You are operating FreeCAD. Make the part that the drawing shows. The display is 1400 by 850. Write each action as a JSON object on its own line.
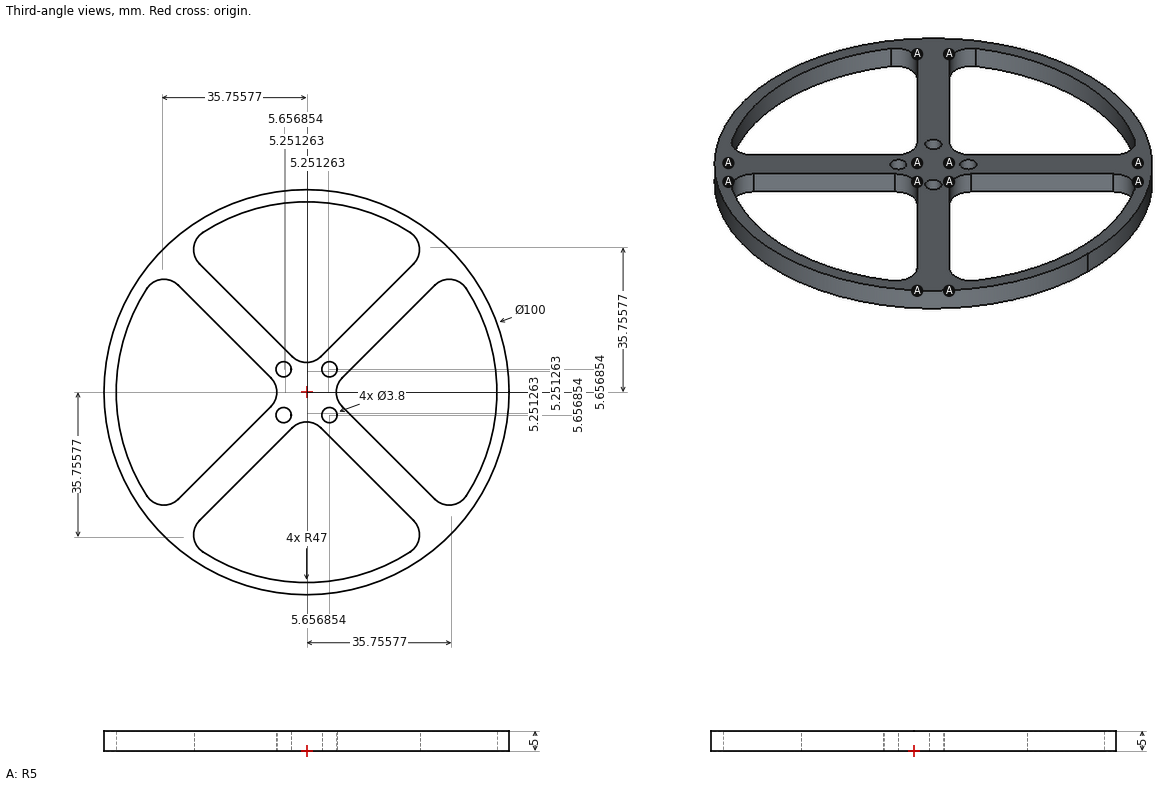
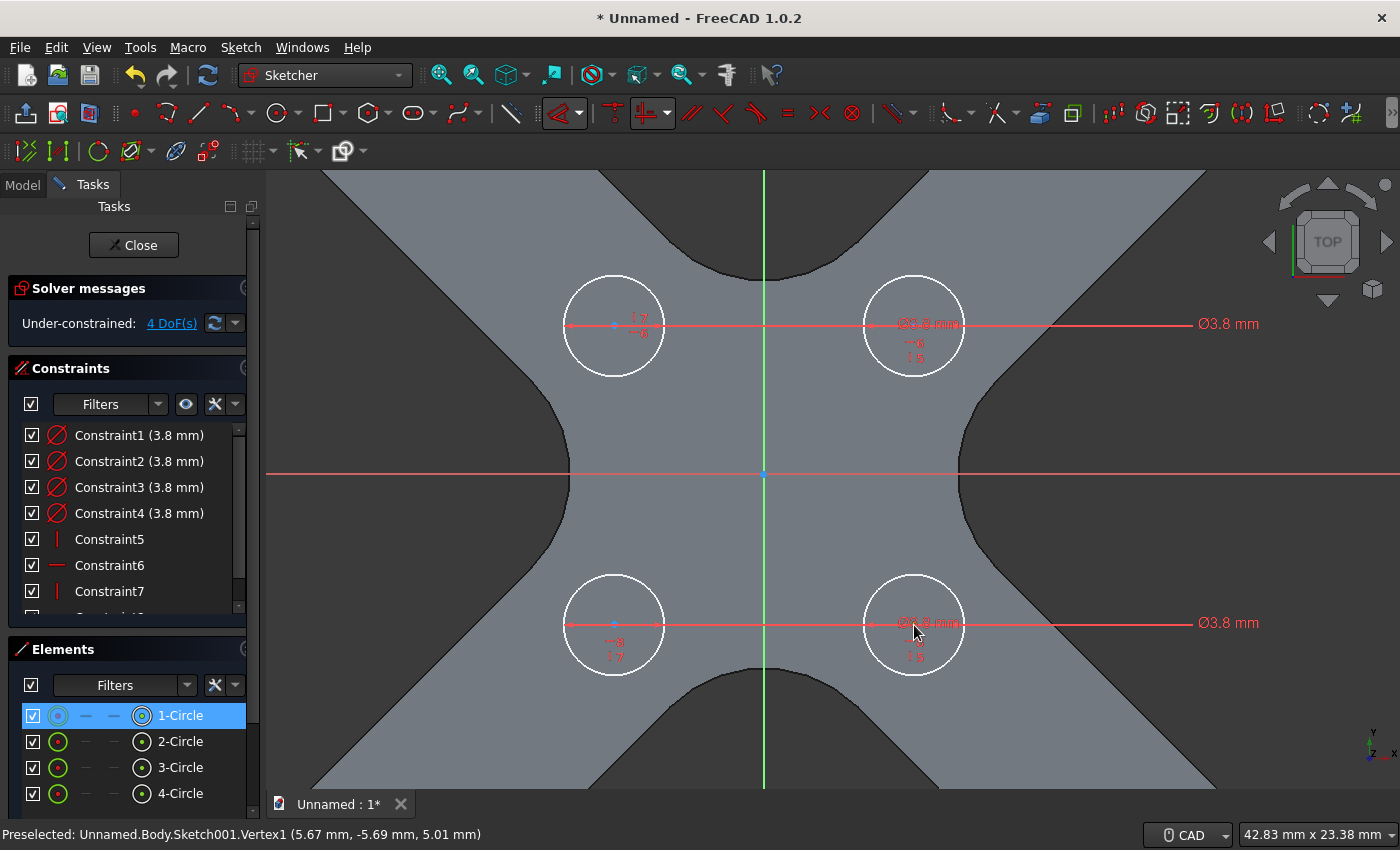
{"action": "left_click", "coordinate": [582, 114]}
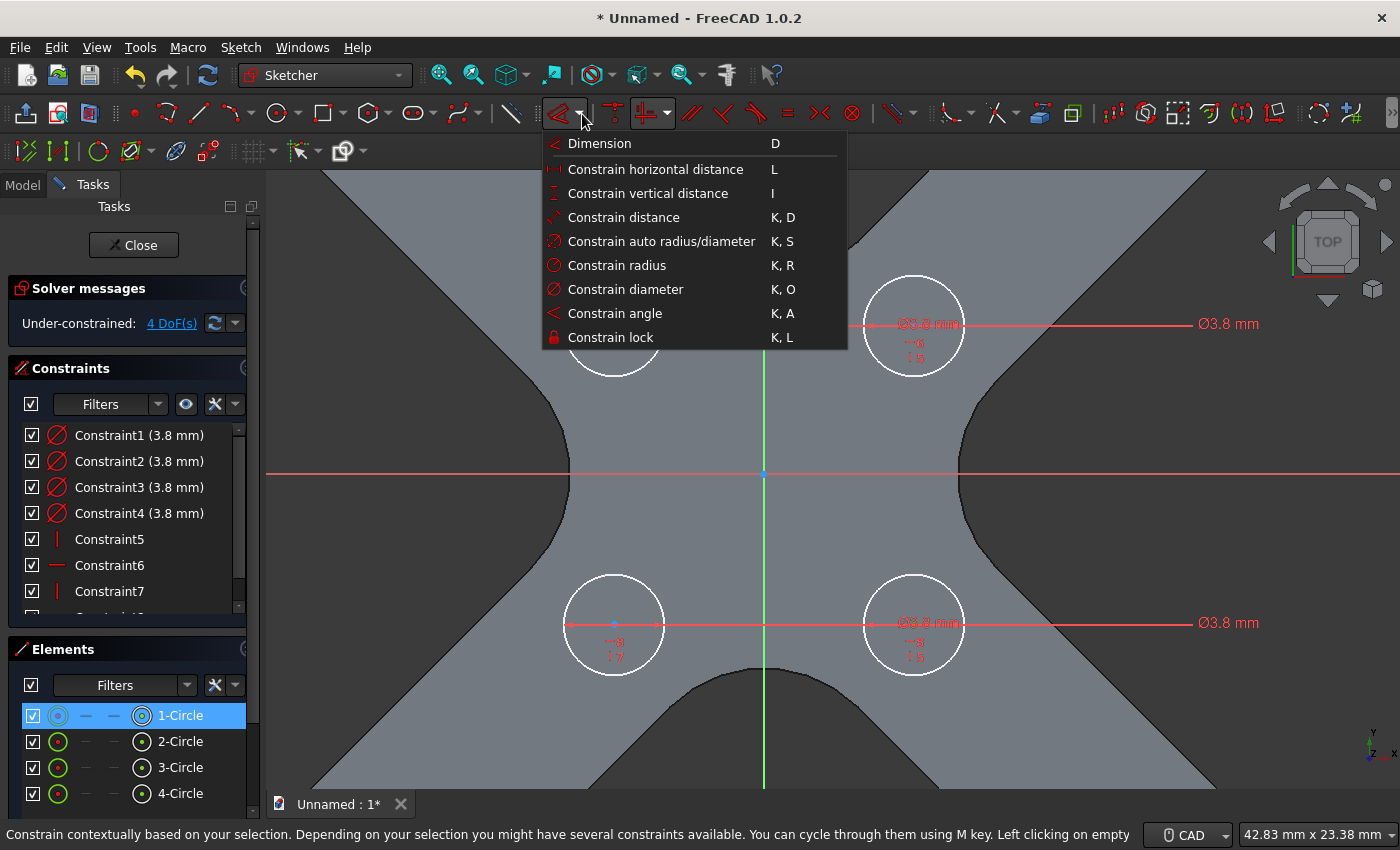
{"action": "left_click", "coordinate": [695, 169]}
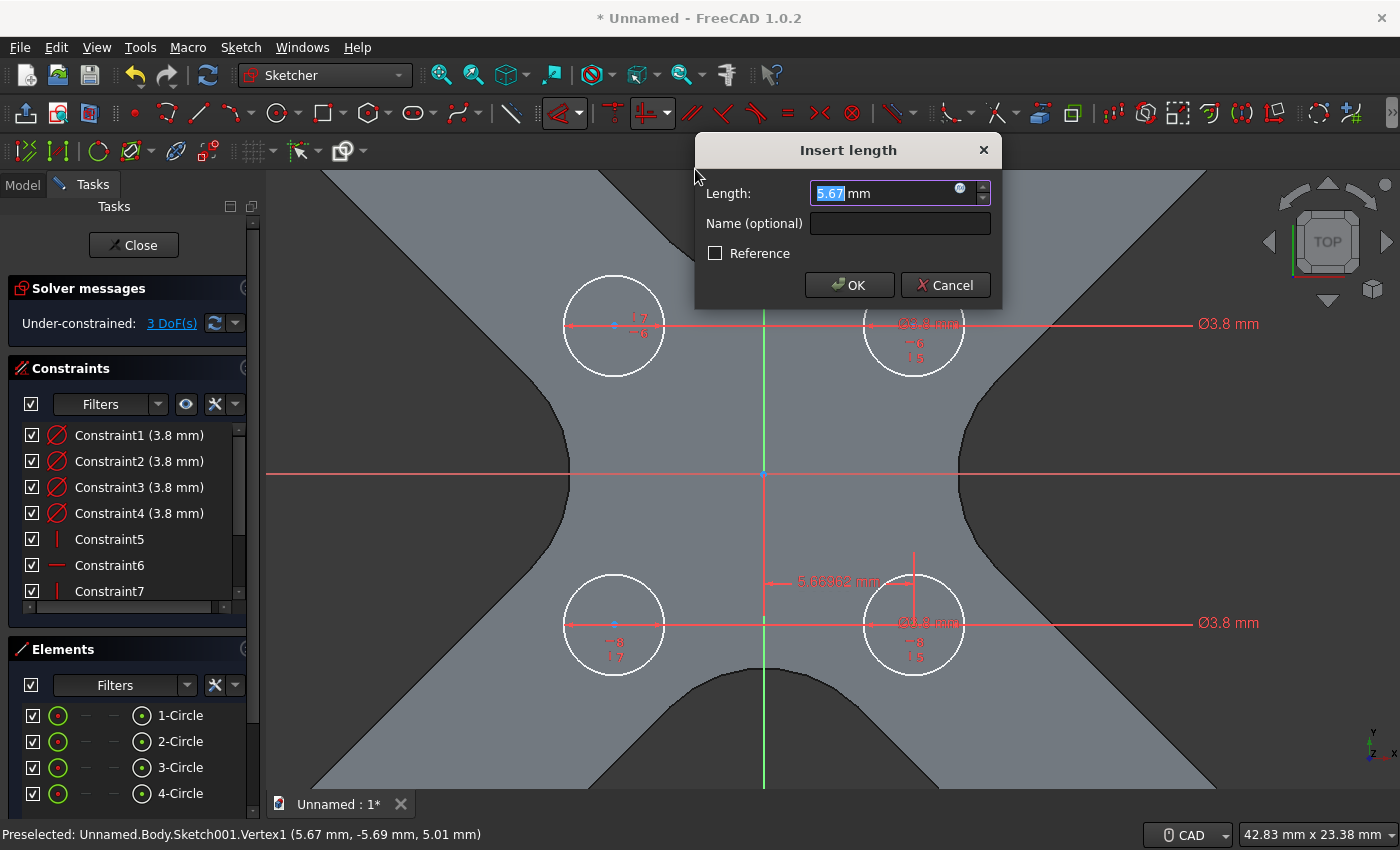
{"action": "type", "text": "5.656854"}
{"action": "key", "text": "Return"}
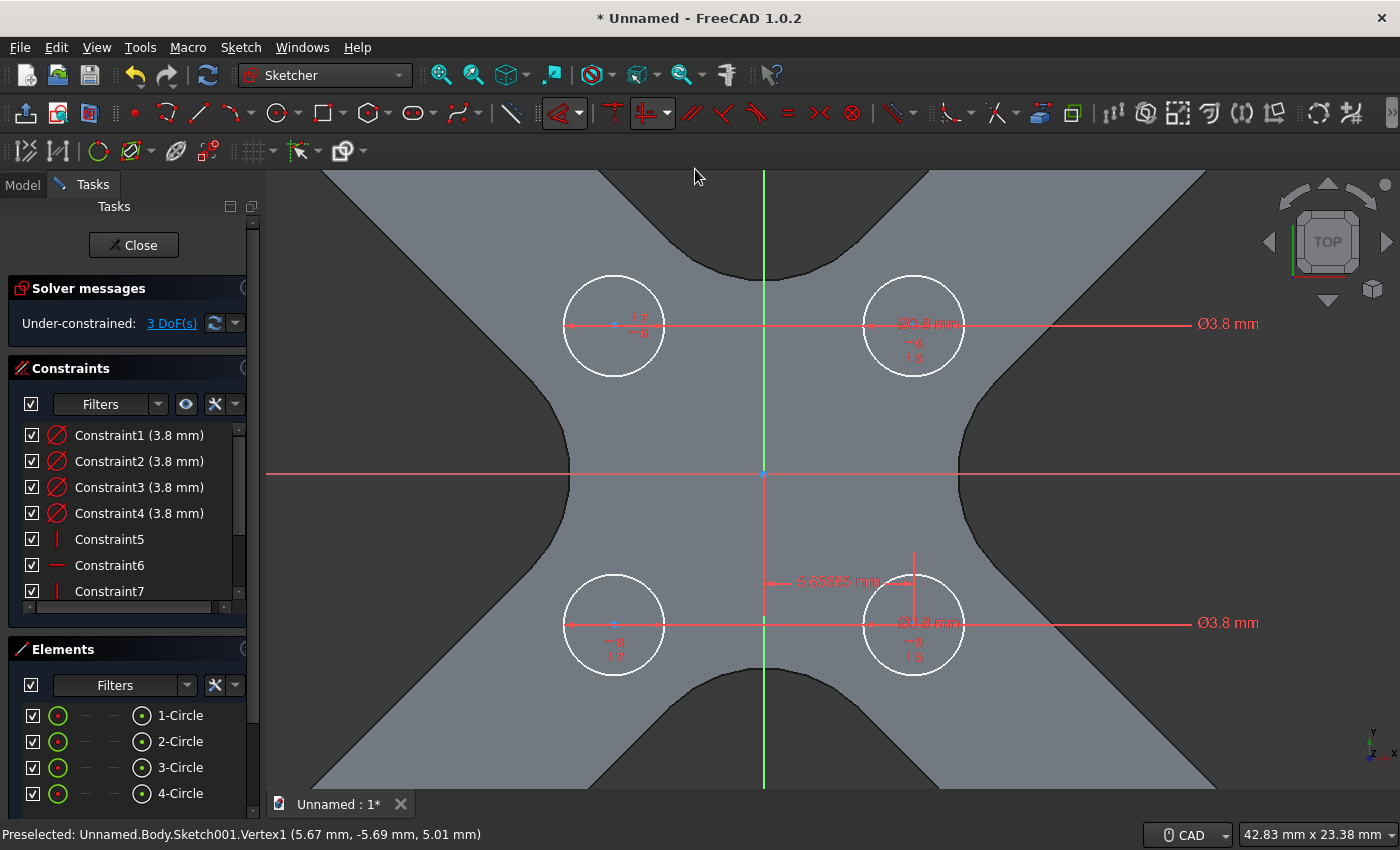
{"action": "left_click", "coordinate": [914, 625]}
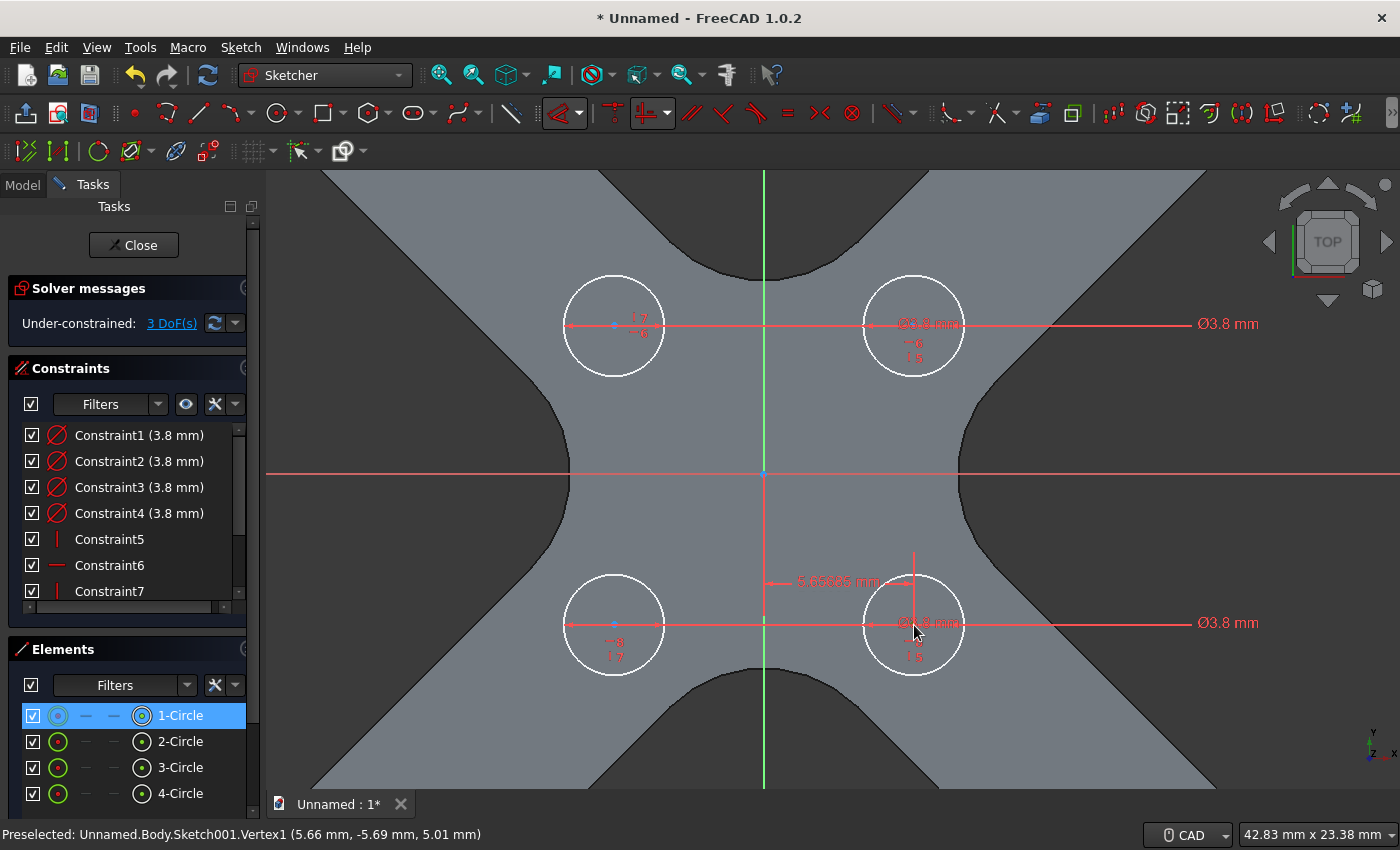
{"action": "left_click", "coordinate": [582, 114]}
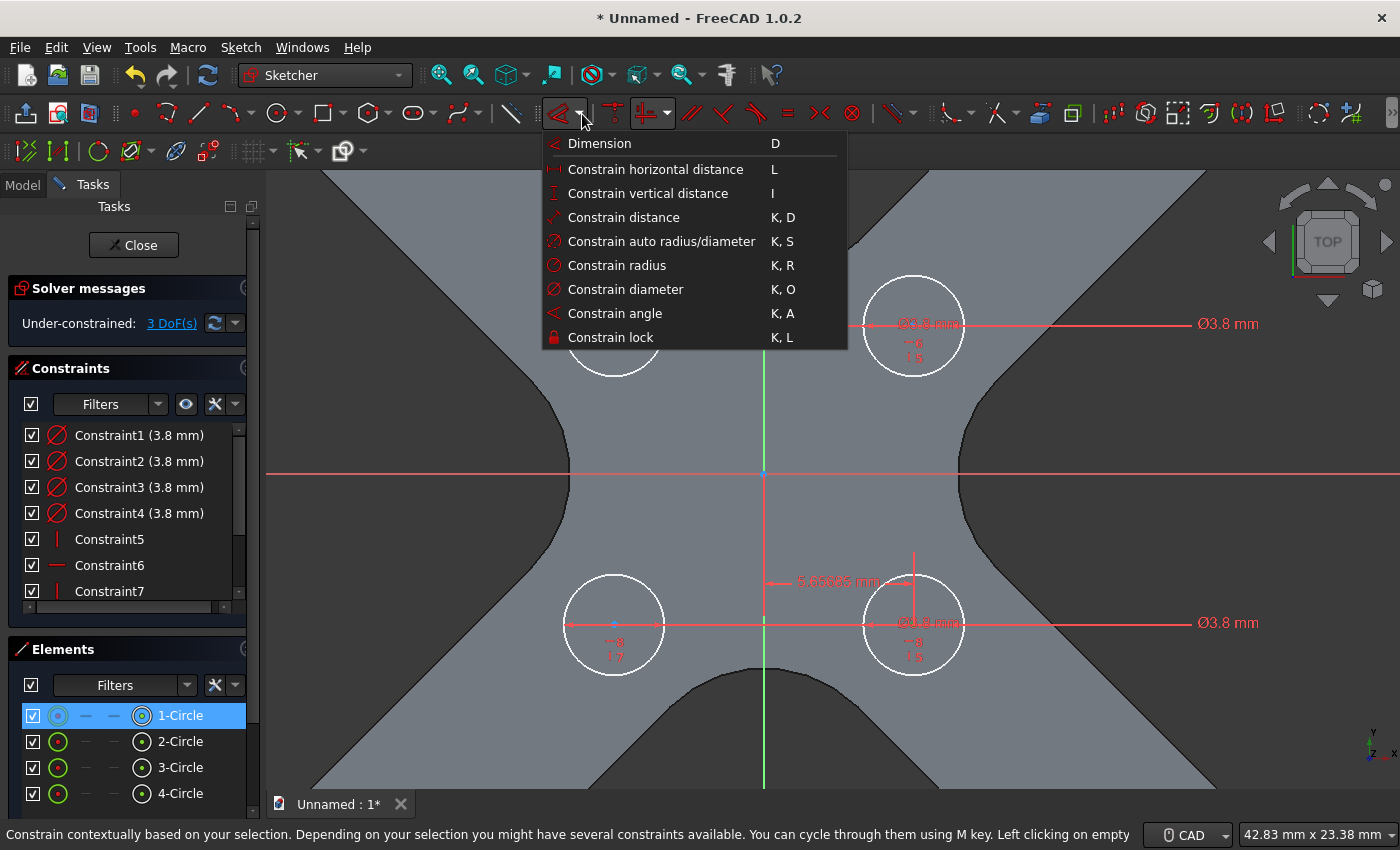
{"action": "left_click", "coordinate": [695, 193]}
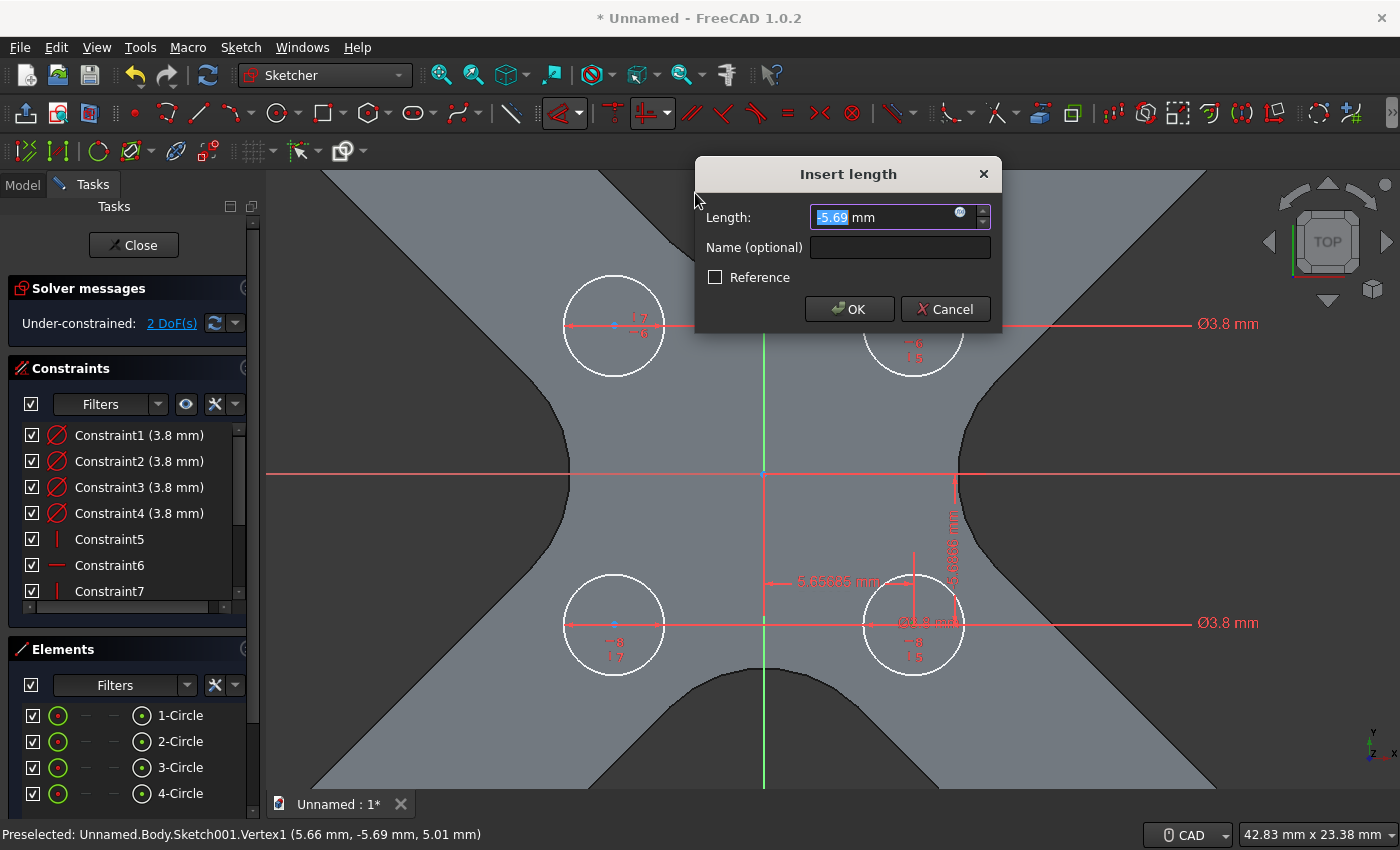
{"action": "type", "text": "-5.656854"}
{"action": "key", "text": "Return"}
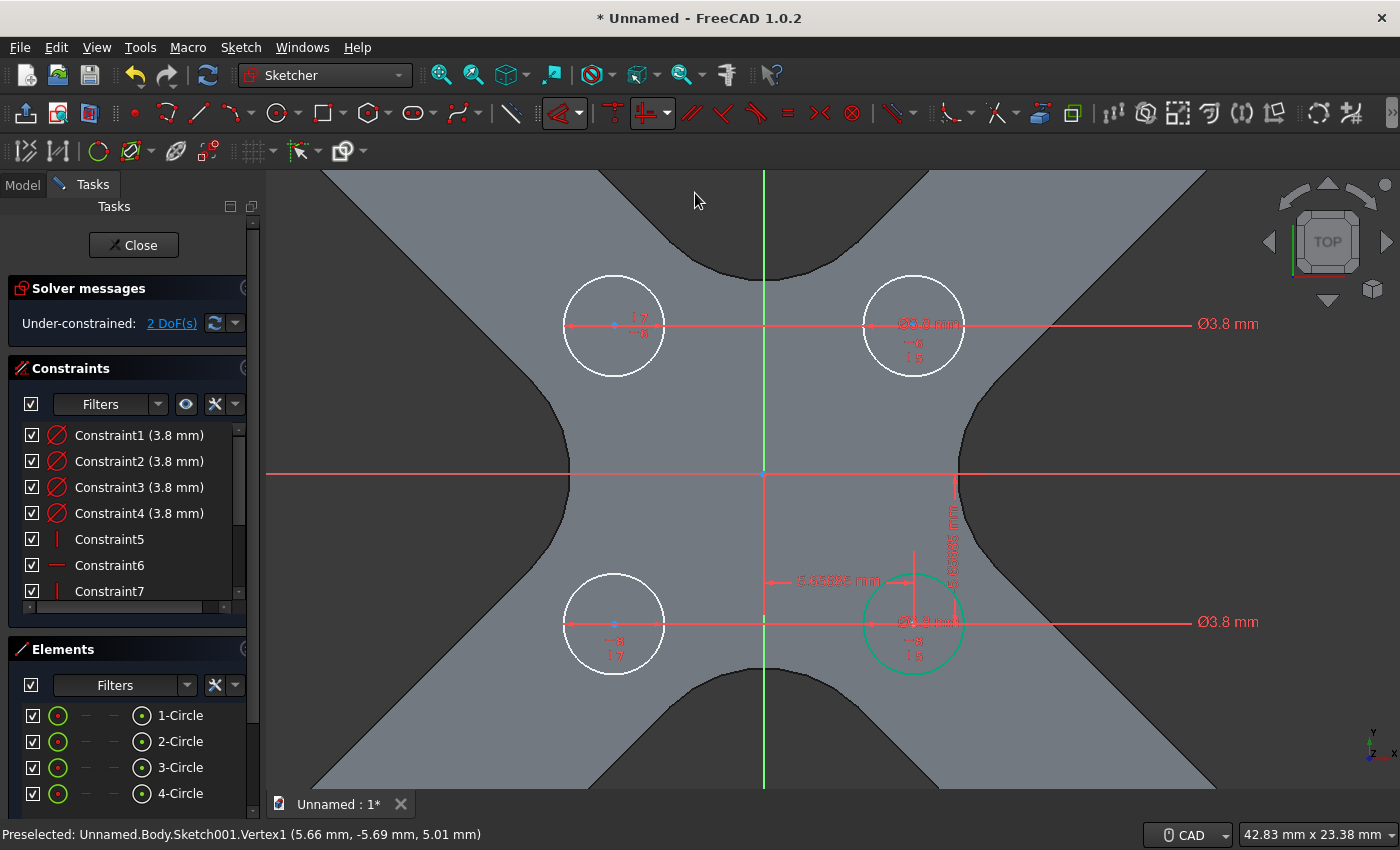
{"action": "left_click", "coordinate": [914, 326]}